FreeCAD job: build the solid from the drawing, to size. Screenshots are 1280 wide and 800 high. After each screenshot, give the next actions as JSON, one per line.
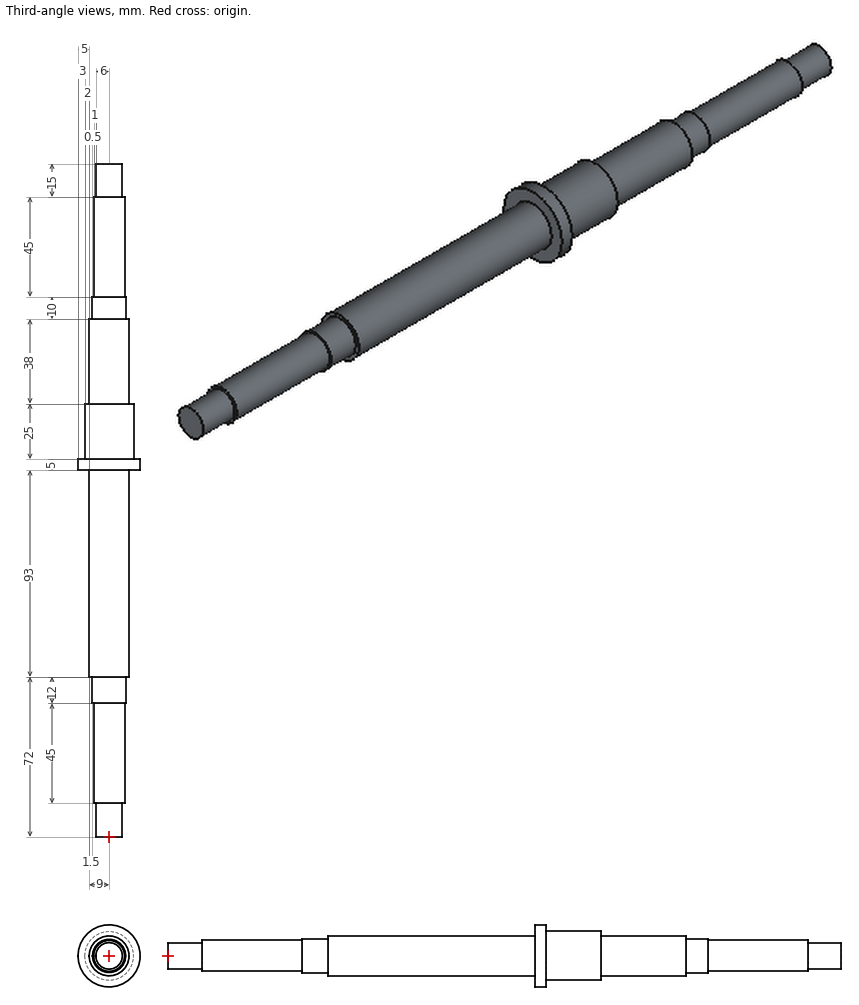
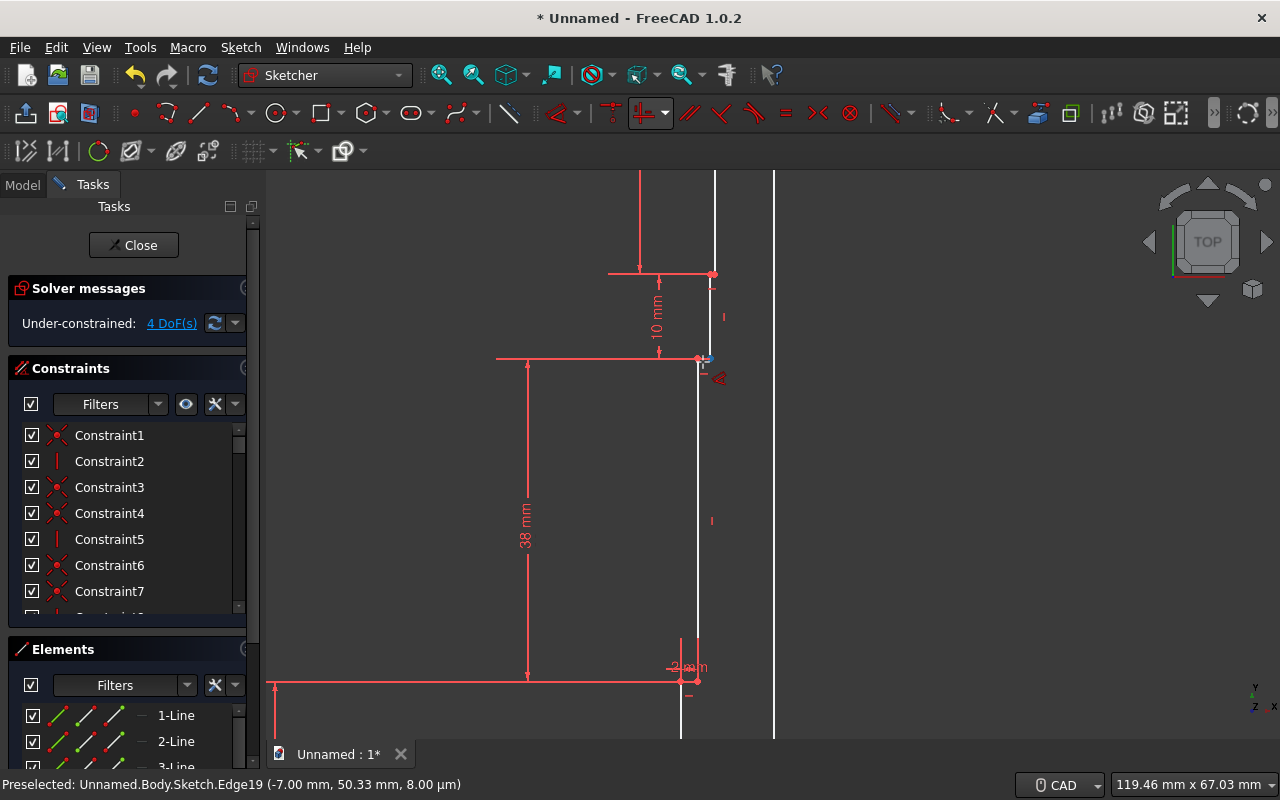
{"action": "left_click", "coordinate": [698, 359]}
{"action": "left_click", "coordinate": [736, 325]}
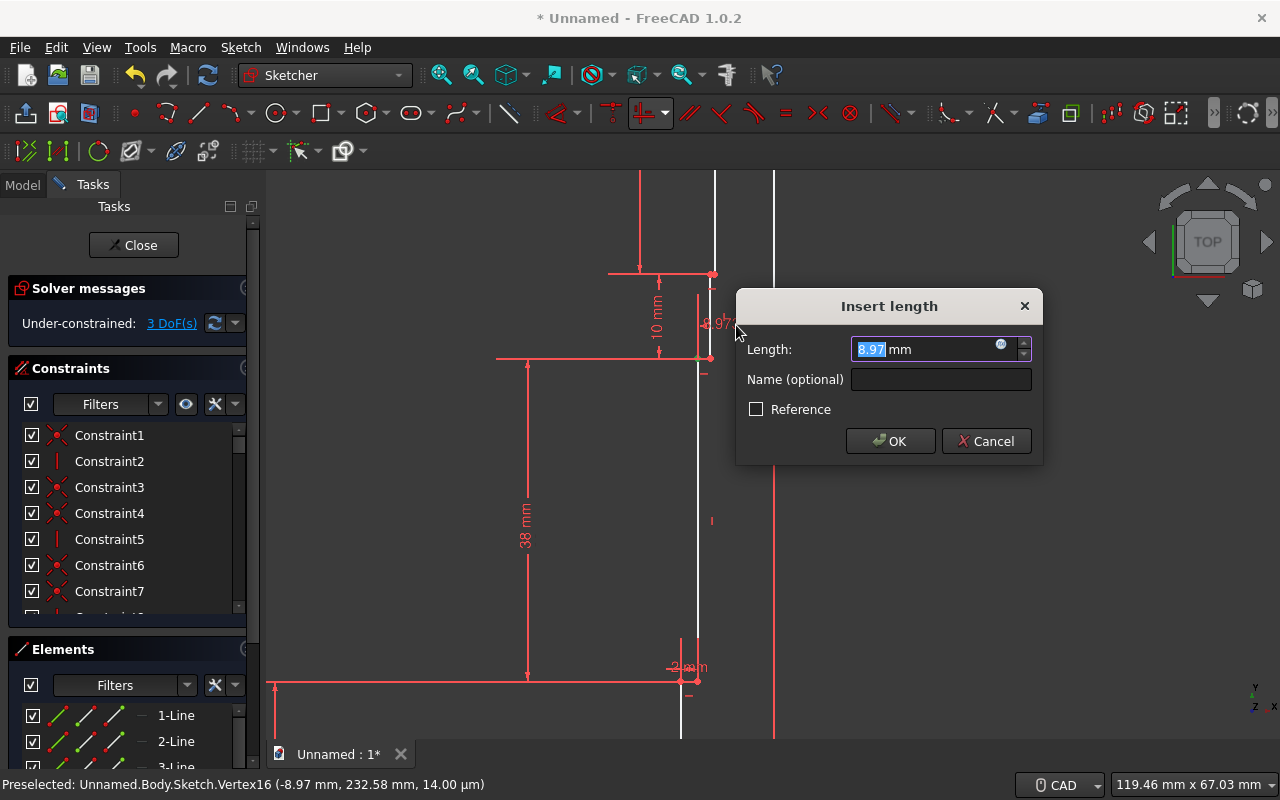
{"action": "type", "text": "9"}
{"action": "key", "text": "Return"}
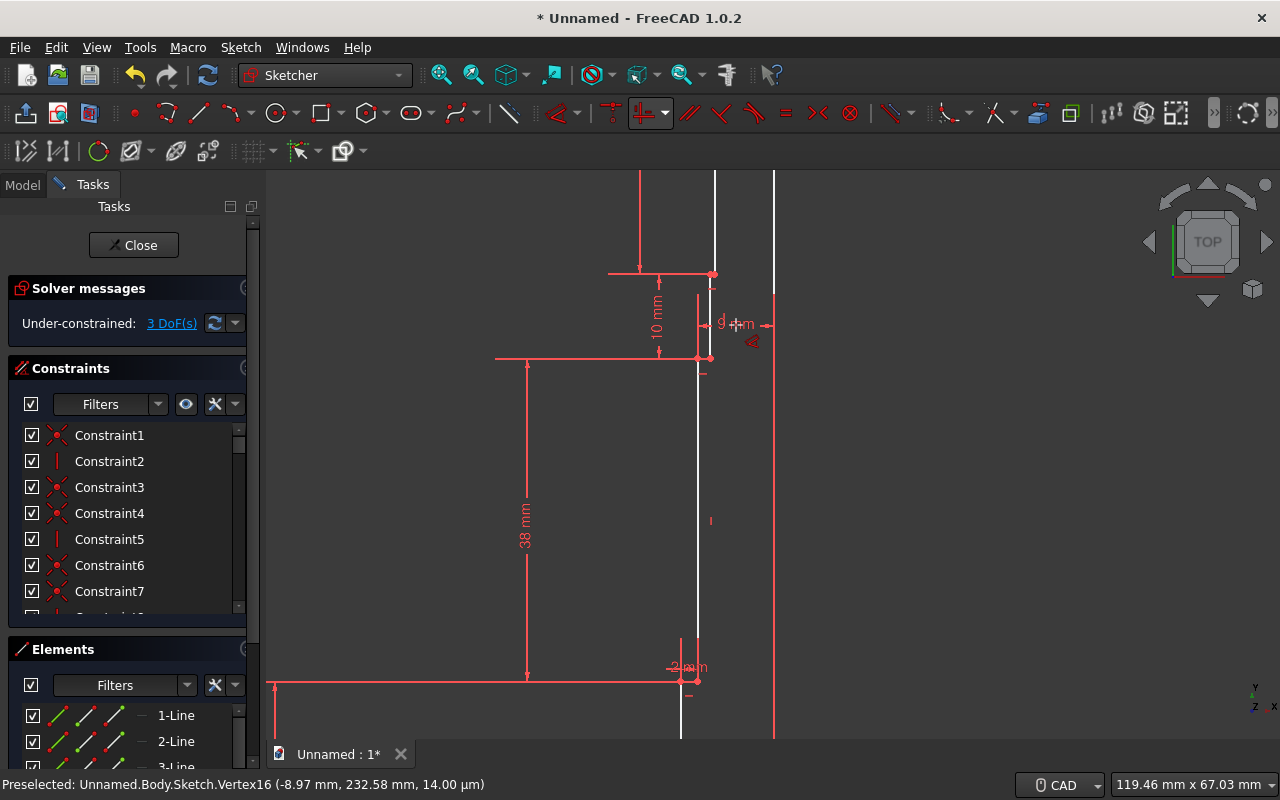
{"action": "scroll", "coordinate": [712, 274], "scroll_direction": "up", "scroll_amount": 12}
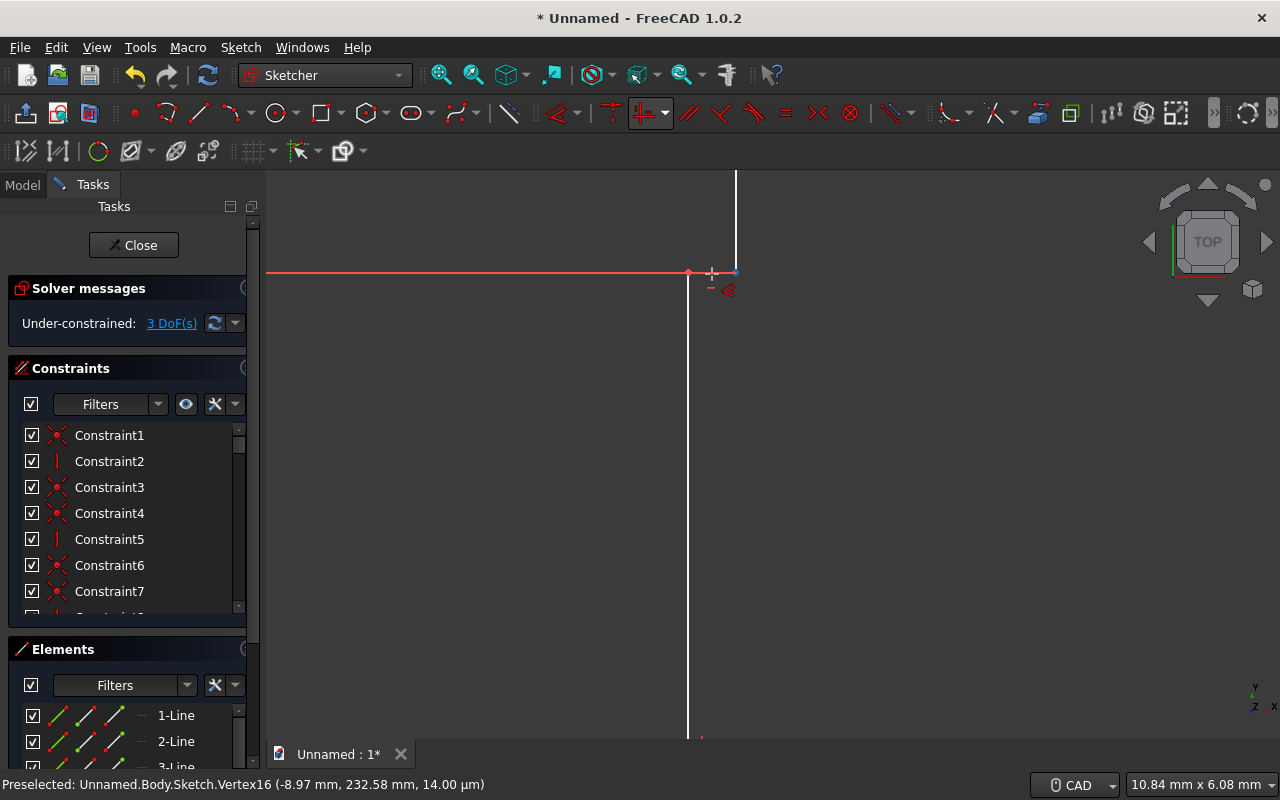
{"action": "left_click", "coordinate": [712, 273]}
{"action": "left_click", "coordinate": [712, 239]}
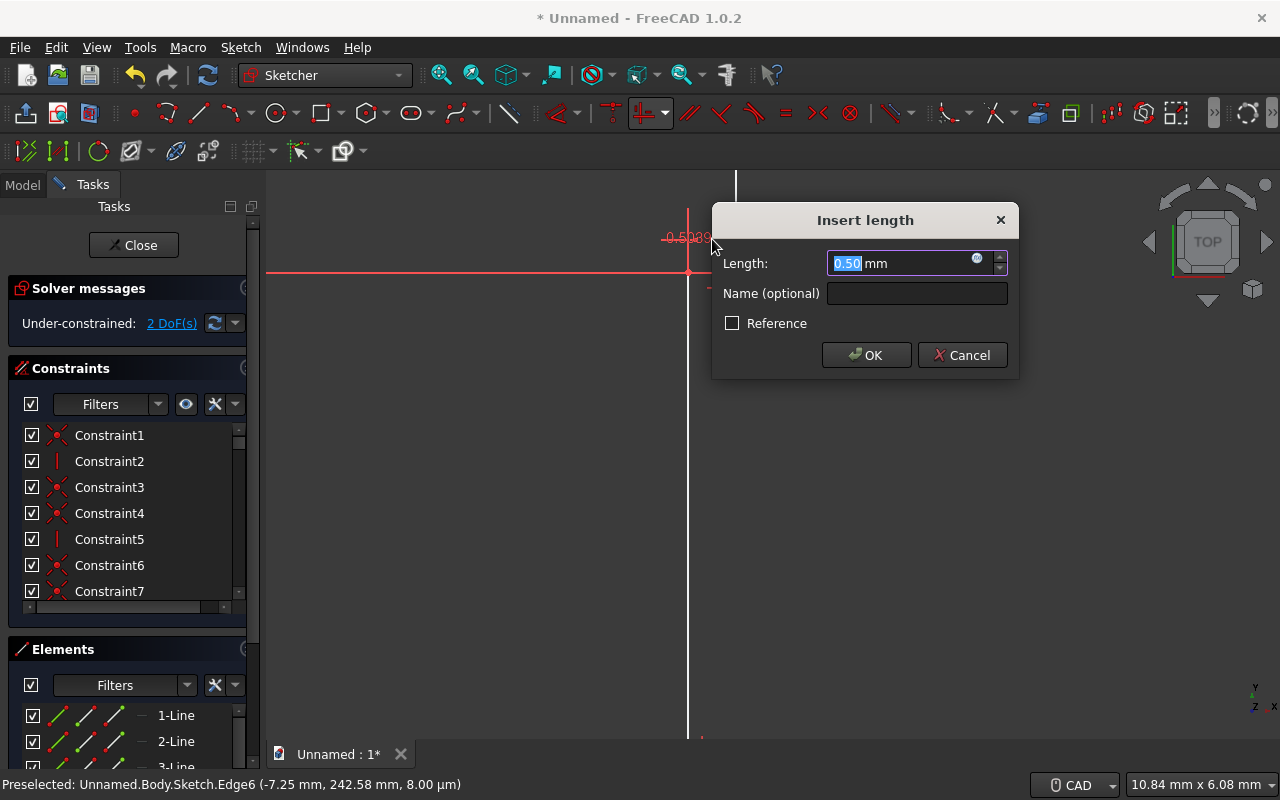
{"action": "type", "text": "0.5"}
{"action": "key", "text": "Return"}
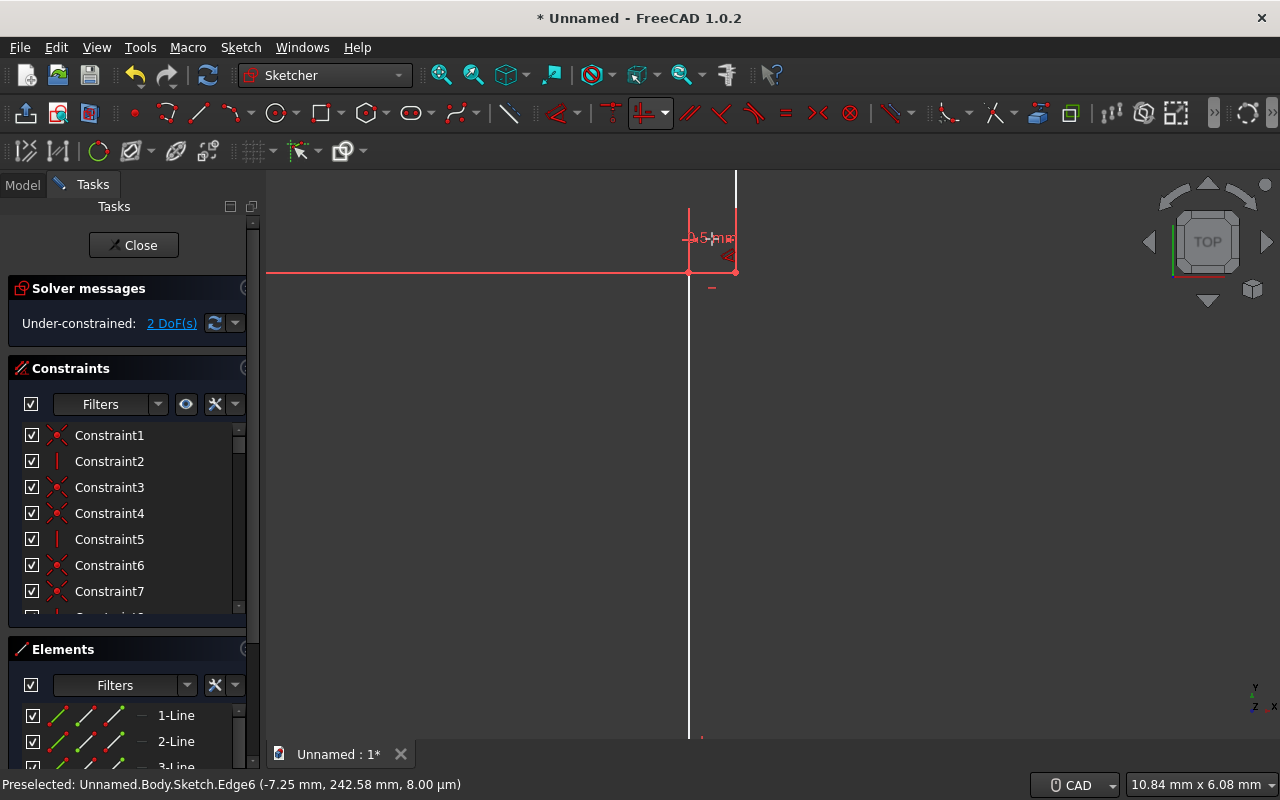
{"action": "scroll", "coordinate": [704, 454], "scroll_direction": "down", "scroll_amount": 15}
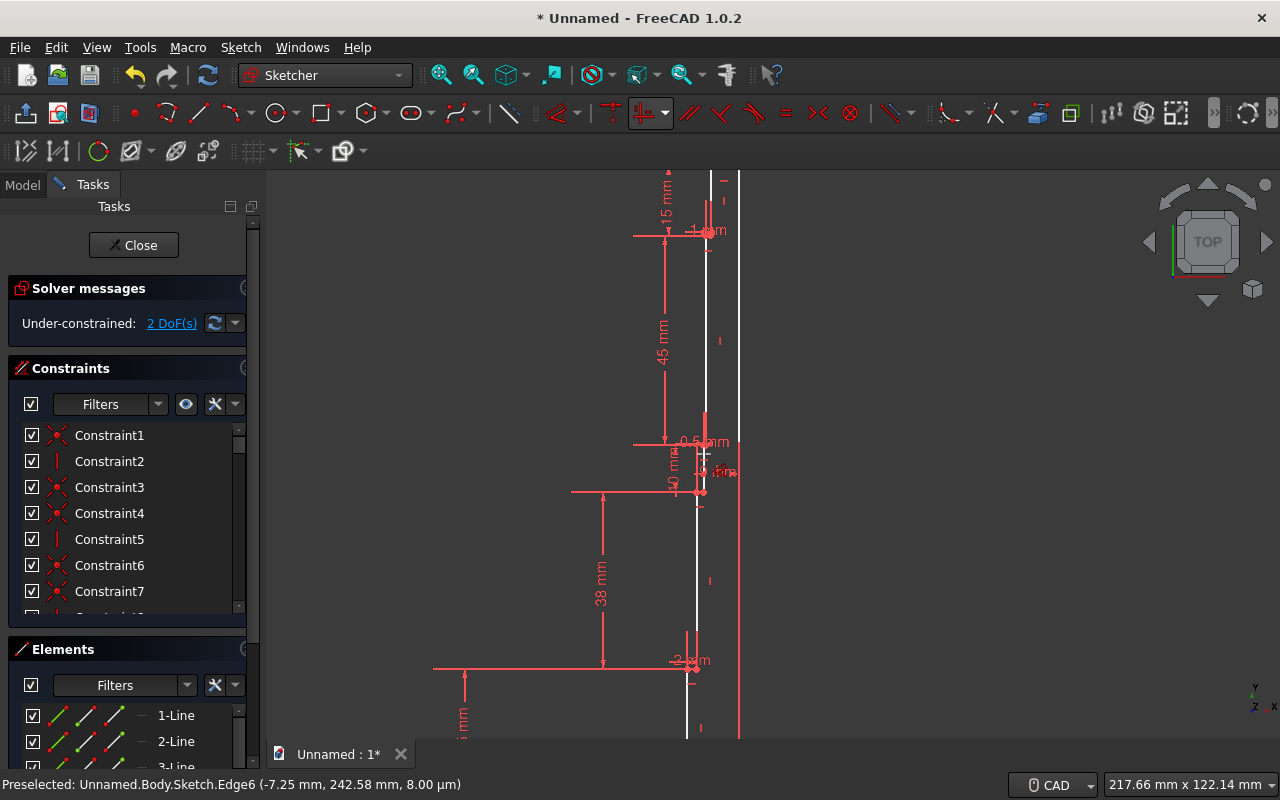
{"action": "scroll", "coordinate": [704, 319], "scroll_direction": "down", "scroll_amount": 7}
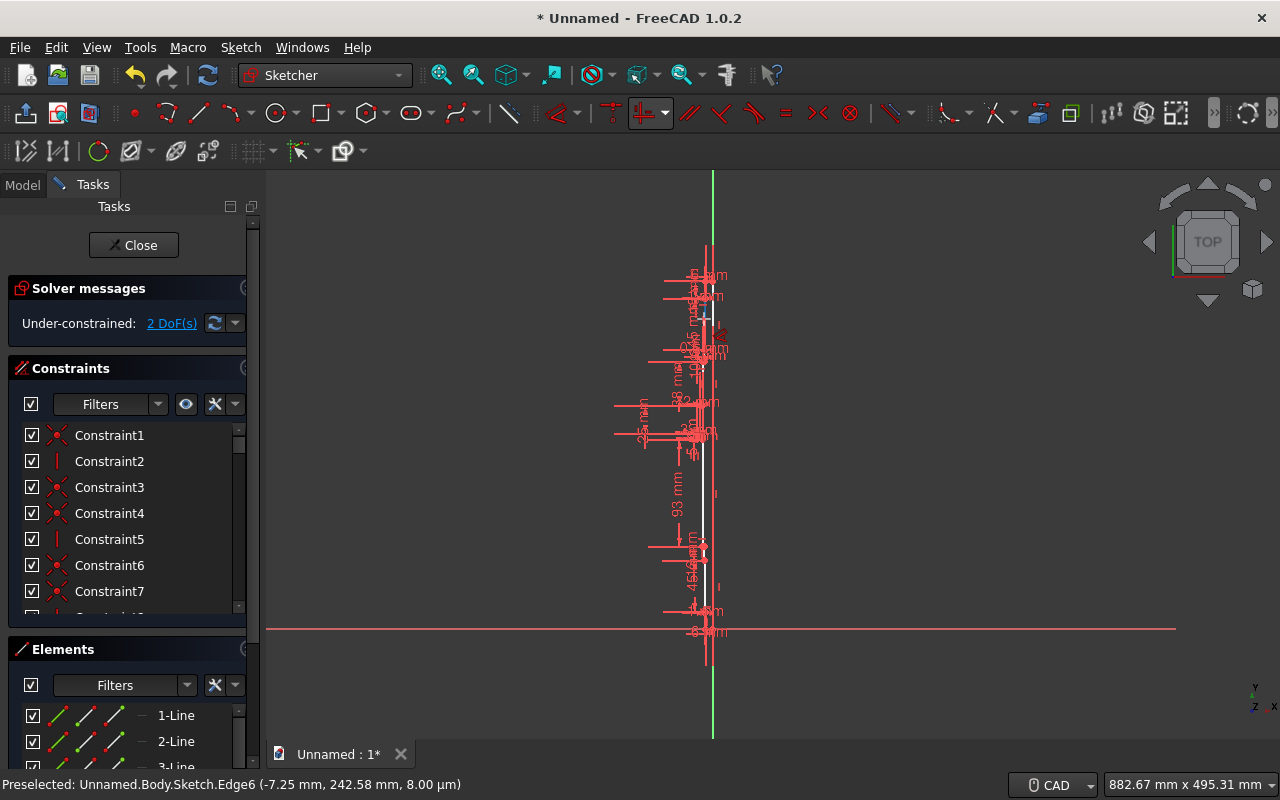
{"action": "scroll", "coordinate": [703, 547], "scroll_direction": "up", "scroll_amount": 16}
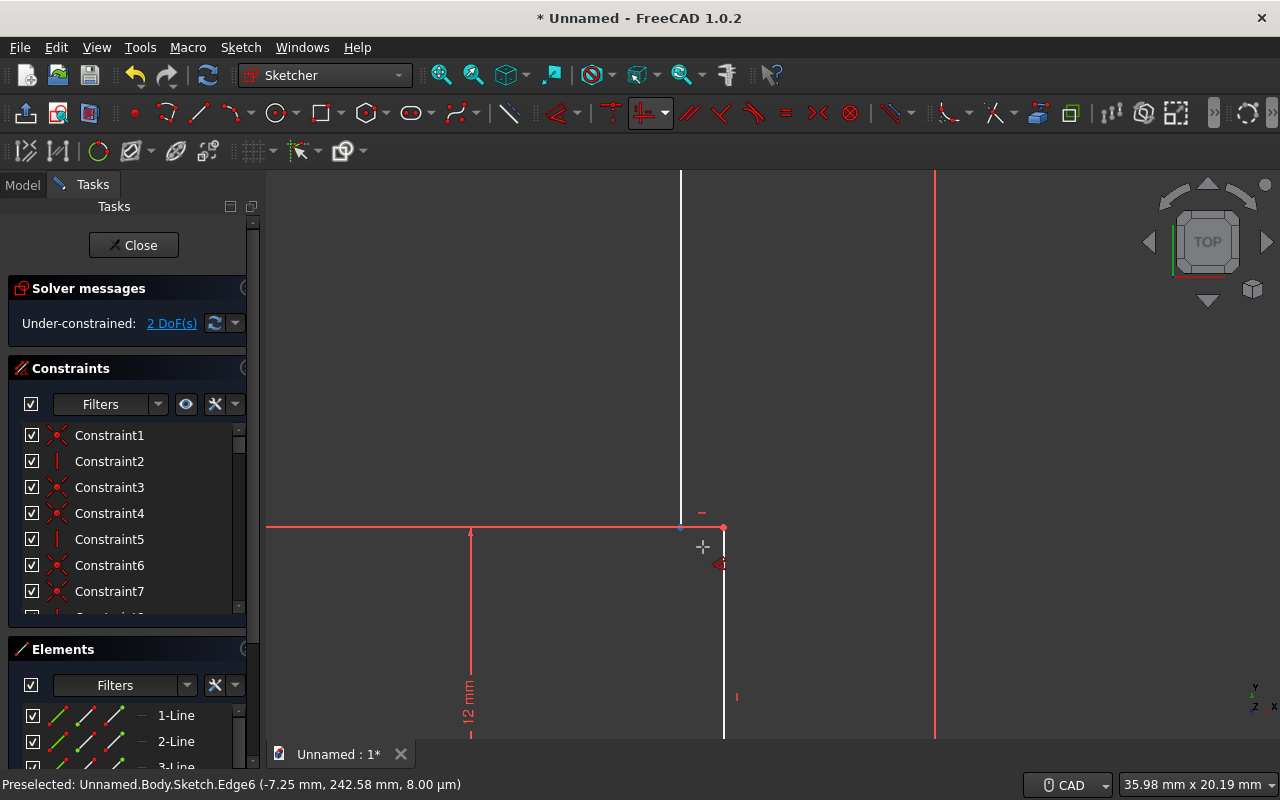
{"action": "left_click", "coordinate": [694, 527]}
{"action": "left_click", "coordinate": [702, 561]}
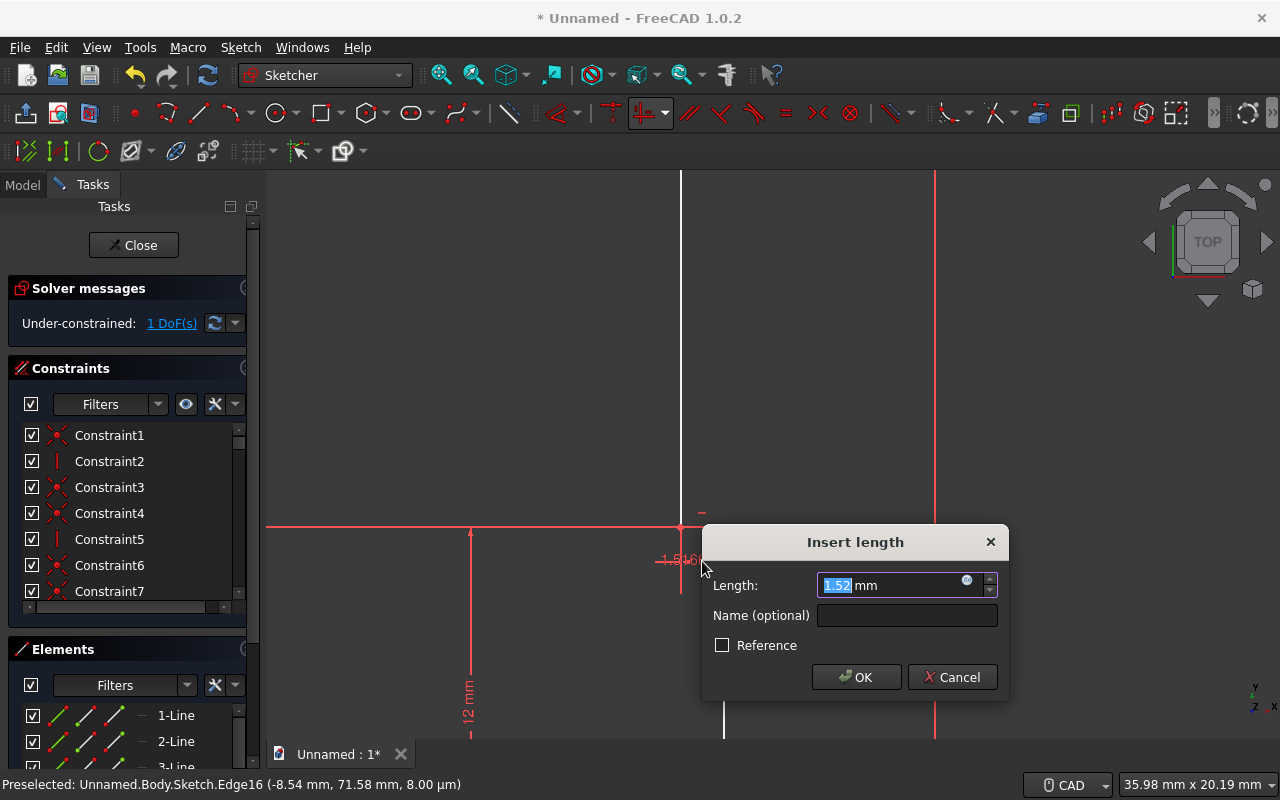
{"action": "type", "text": "1.5"}
{"action": "key", "text": "Return"}